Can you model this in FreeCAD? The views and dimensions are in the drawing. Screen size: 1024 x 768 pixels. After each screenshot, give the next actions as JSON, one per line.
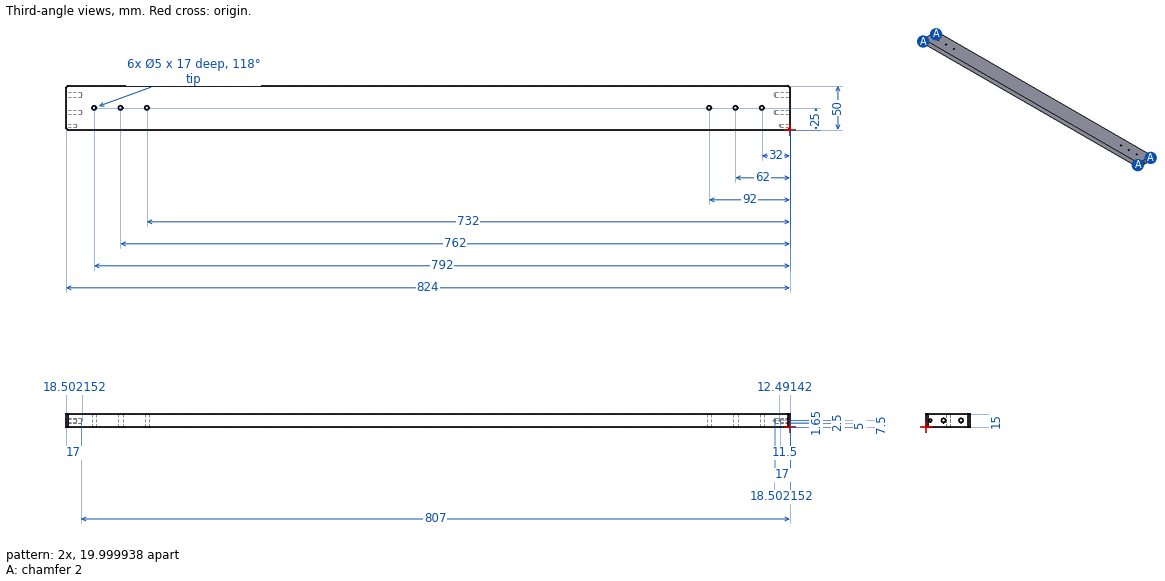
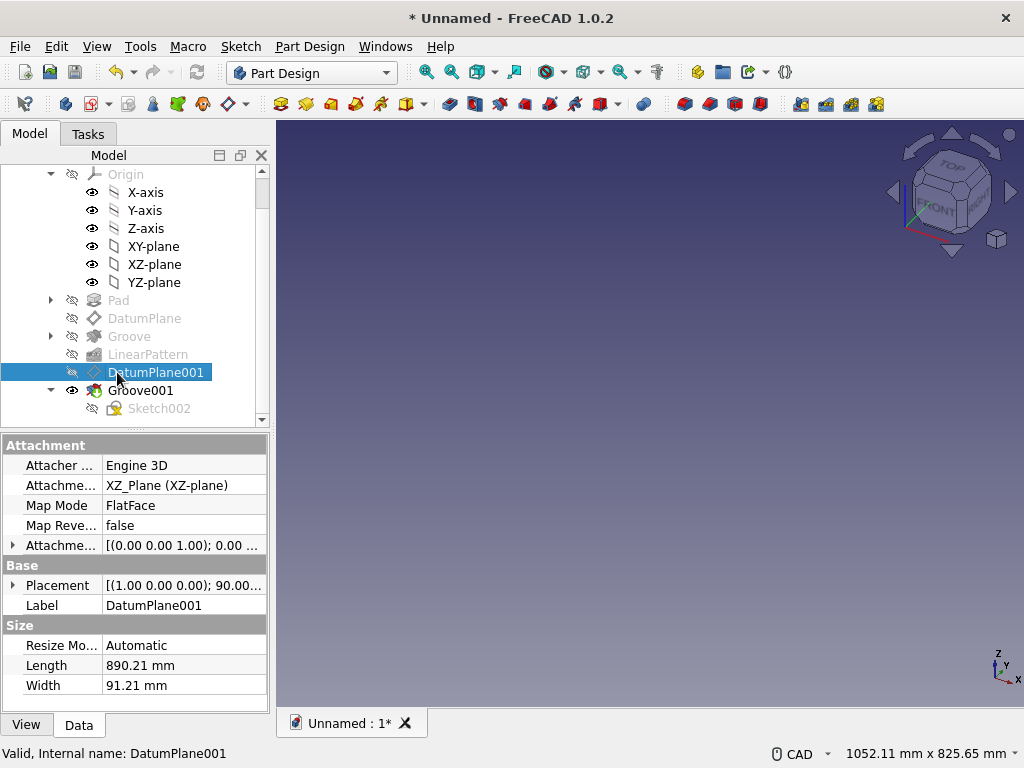
{"action": "left_click", "coordinate": [427, 72]}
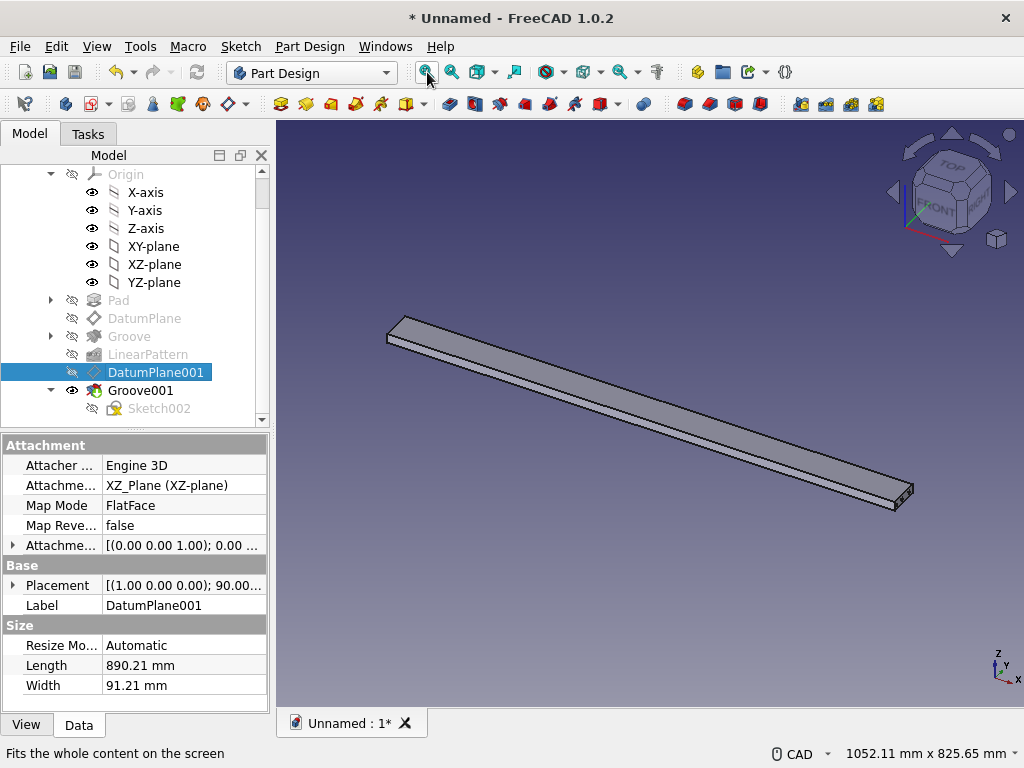
{"action": "left_click", "coordinate": [137, 282]}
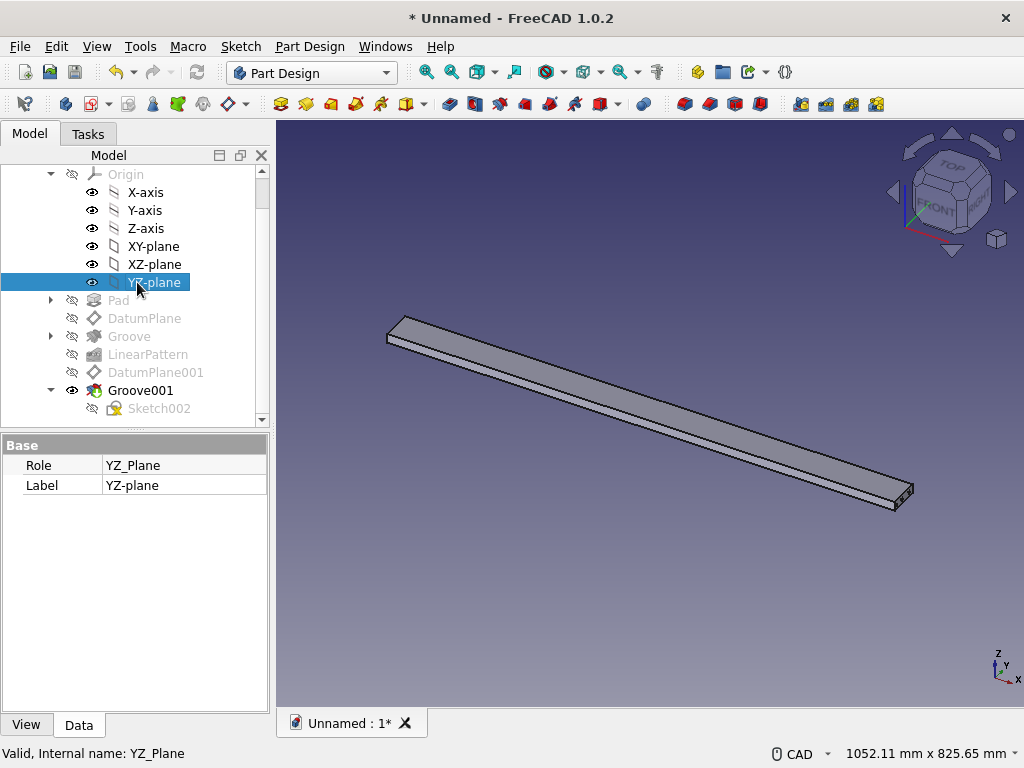
{"action": "left_click", "coordinate": [228, 104]}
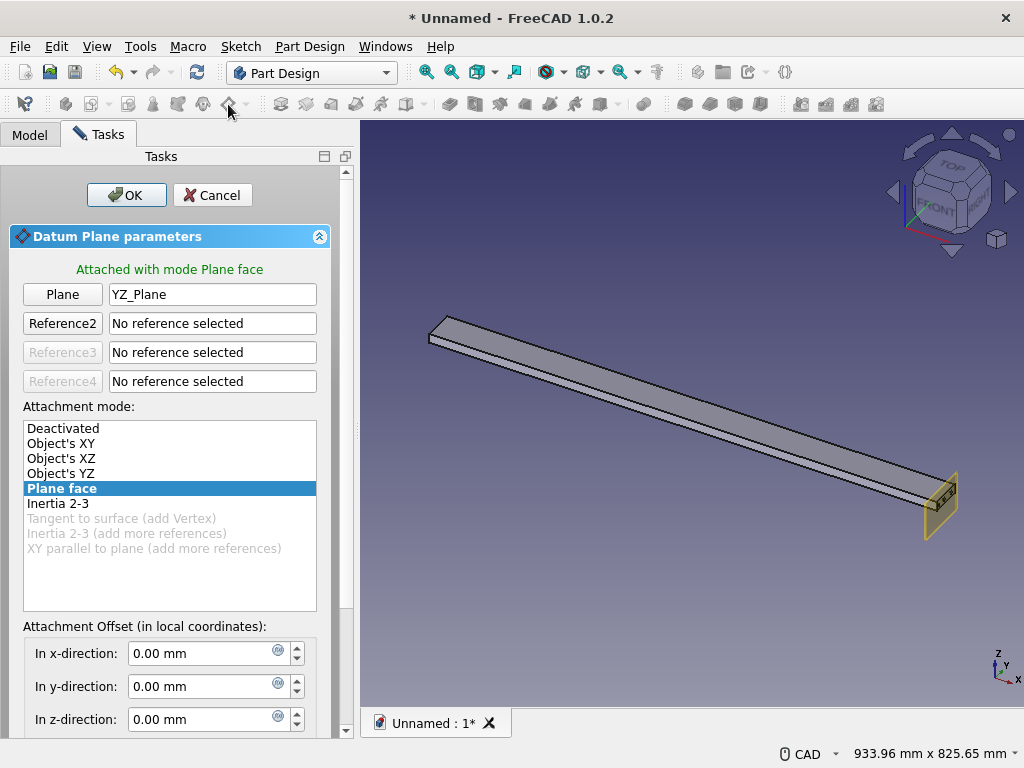
{"action": "triple_click", "coordinate": [210, 720]}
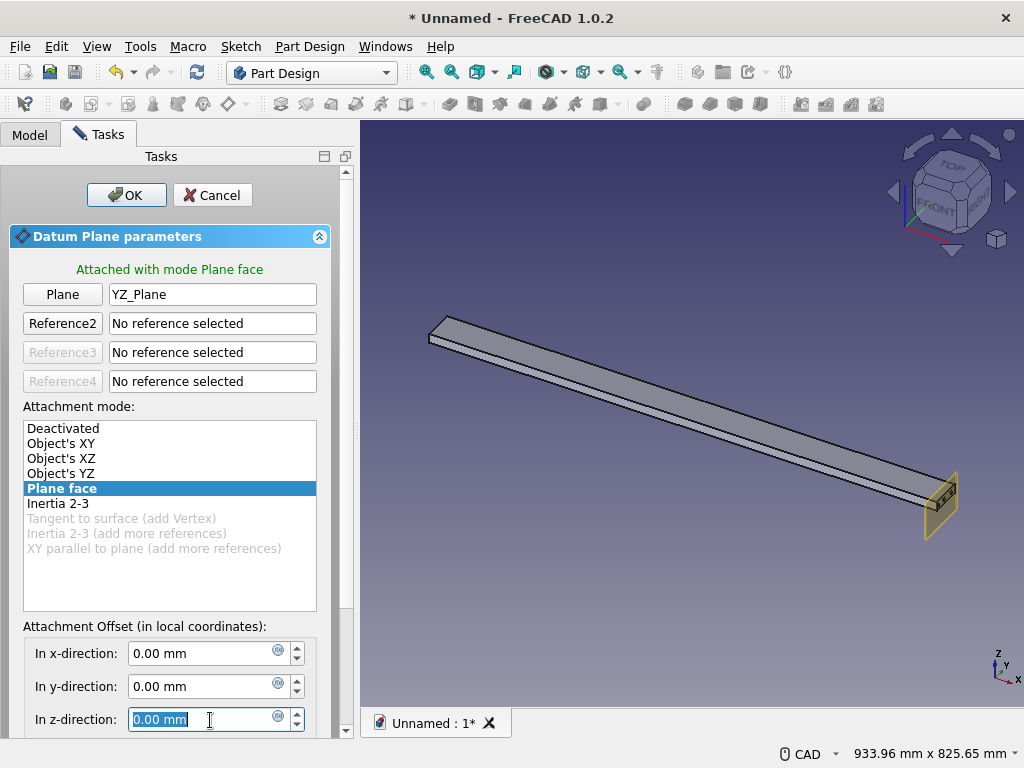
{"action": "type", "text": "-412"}
{"action": "key", "text": "Tab"}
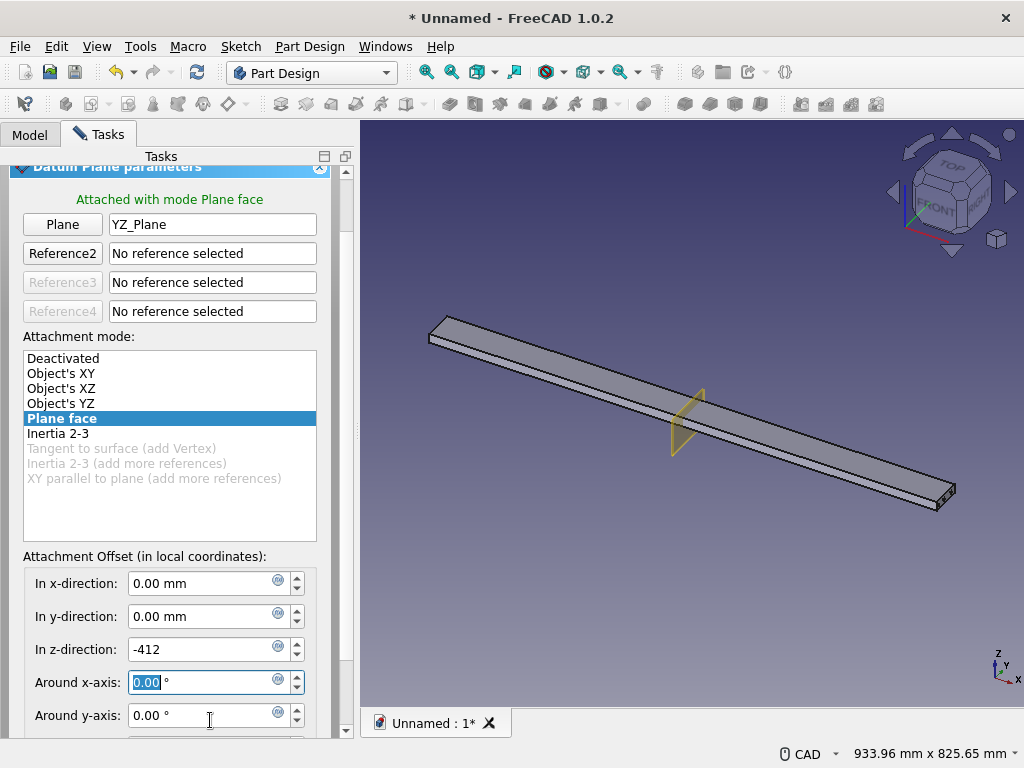
{"action": "scroll", "coordinate": [346, 452], "scroll_direction": "up", "scroll_amount": 2}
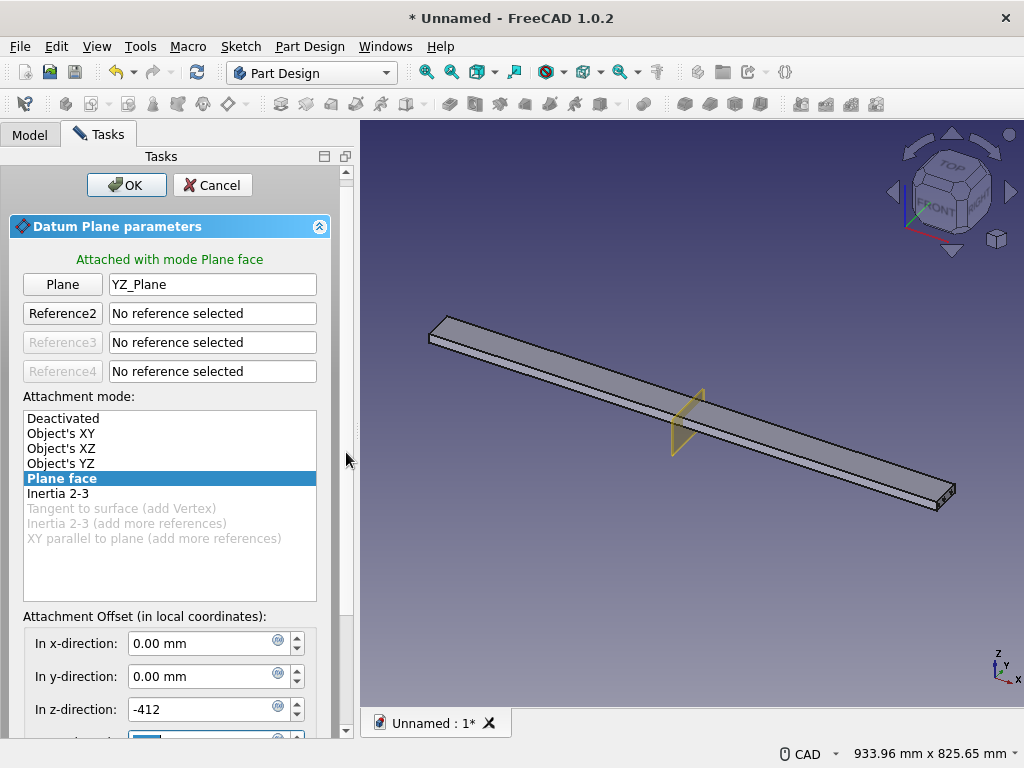
{"action": "left_click", "coordinate": [127, 195]}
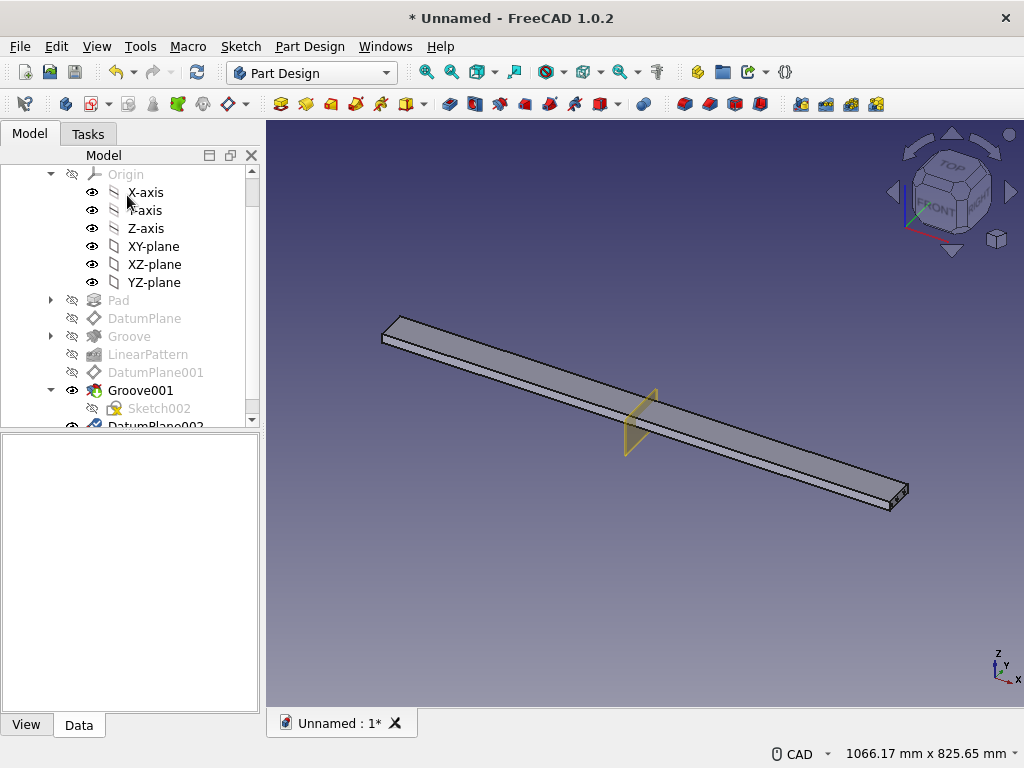
{"action": "left_click", "coordinate": [117, 336]}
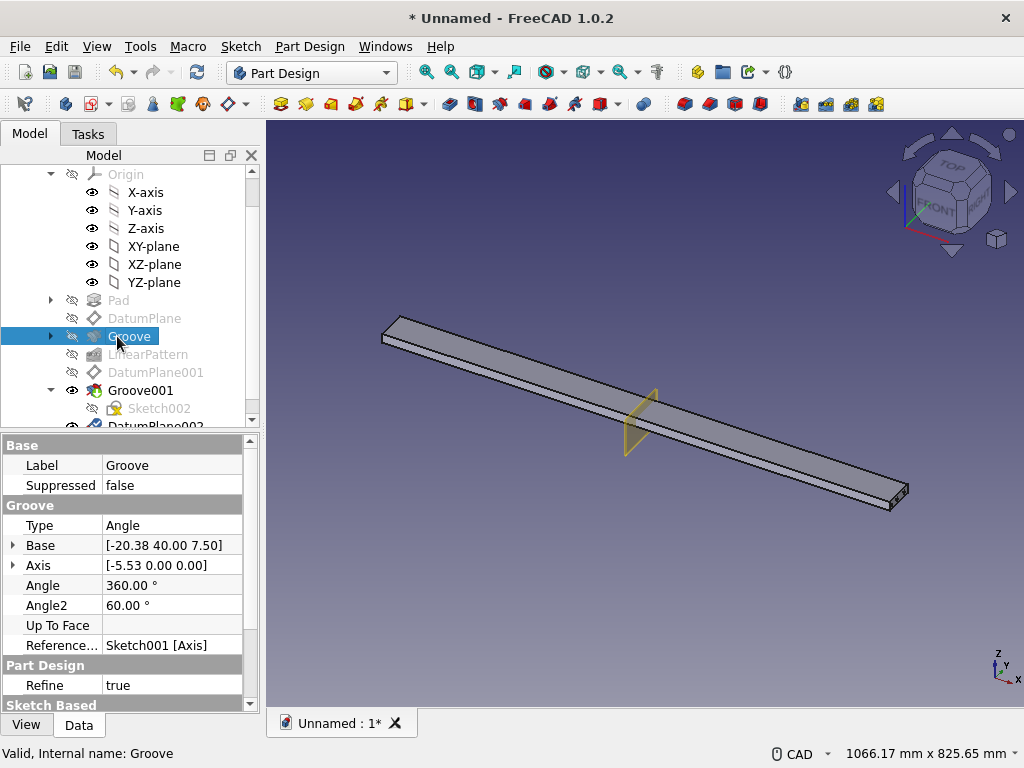
{"action": "left_click", "coordinate": [117, 390], "text": "ctrl"}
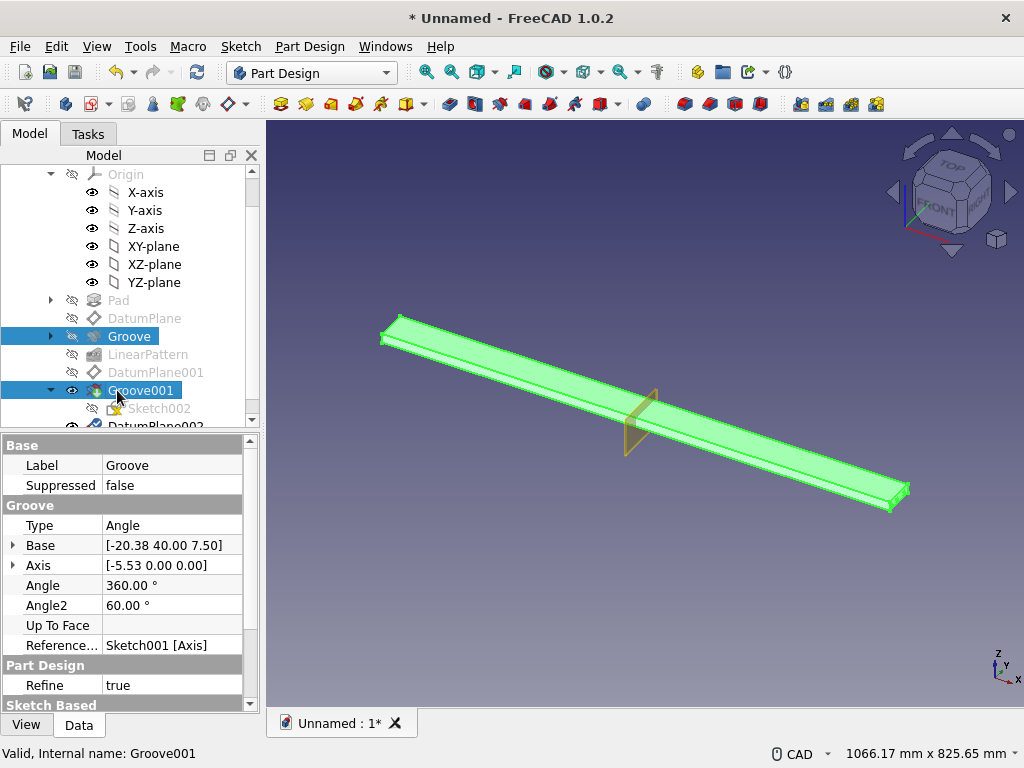
{"action": "left_click", "coordinate": [801, 104]}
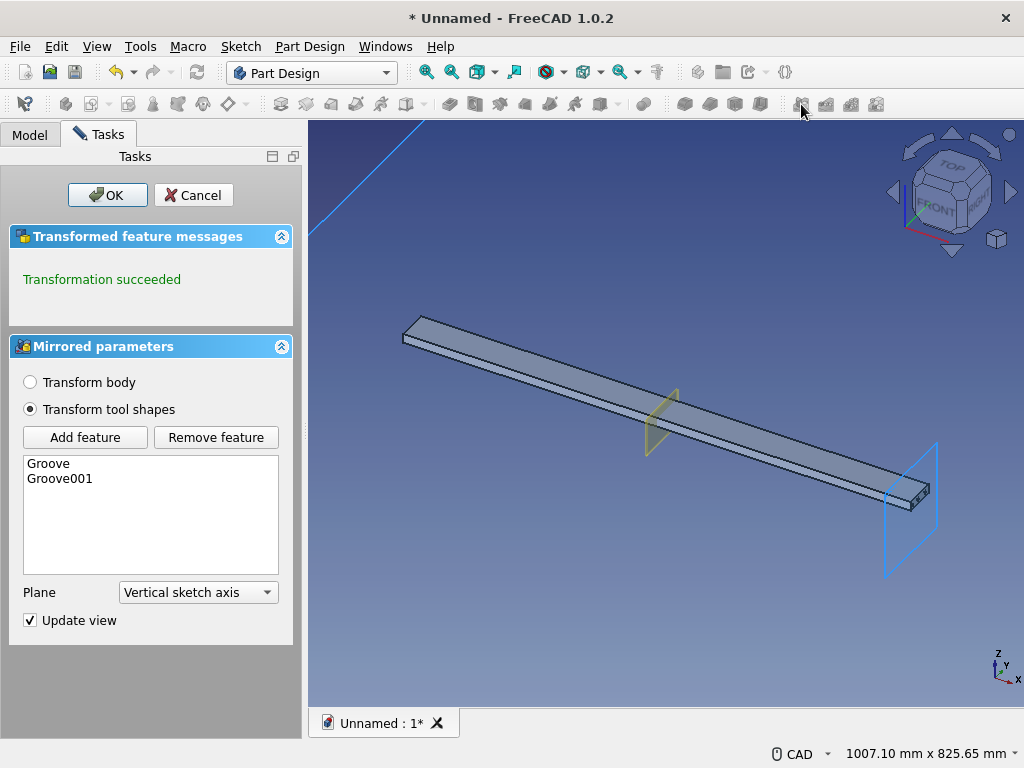
{"action": "left_click", "coordinate": [199, 592]}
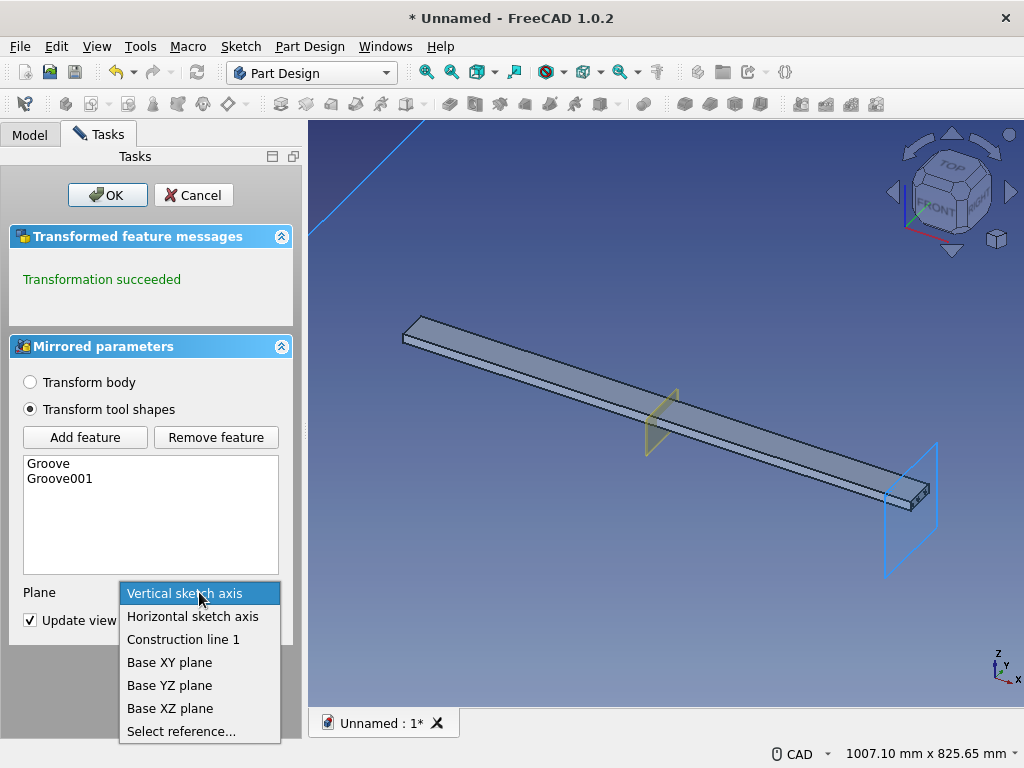
{"action": "left_click", "coordinate": [198, 732]}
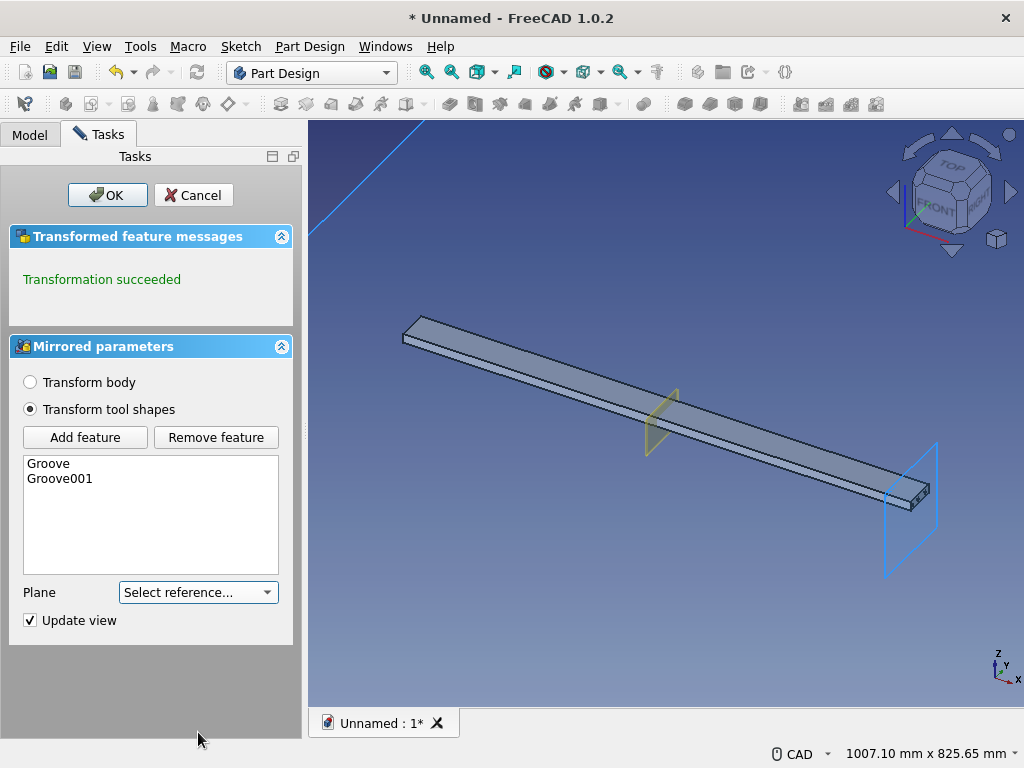
{"action": "left_click", "coordinate": [30, 134]}